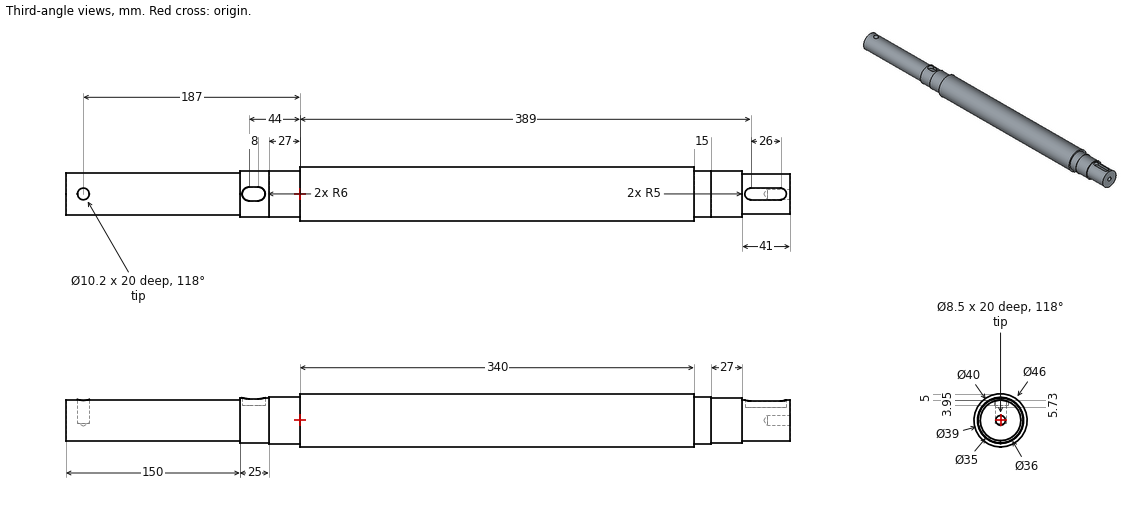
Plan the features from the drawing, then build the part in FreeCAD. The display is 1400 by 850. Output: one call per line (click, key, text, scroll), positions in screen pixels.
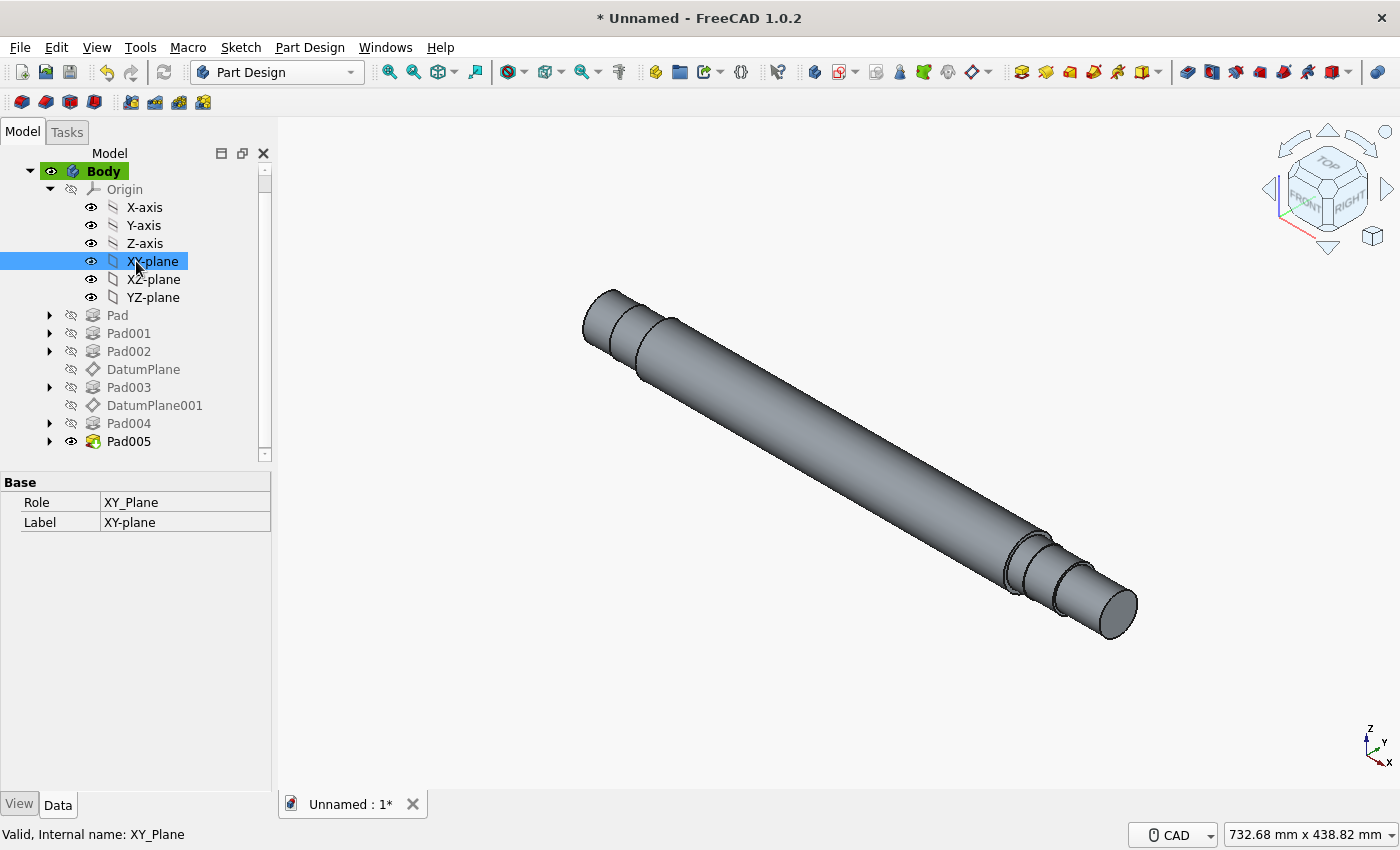
click(972, 72)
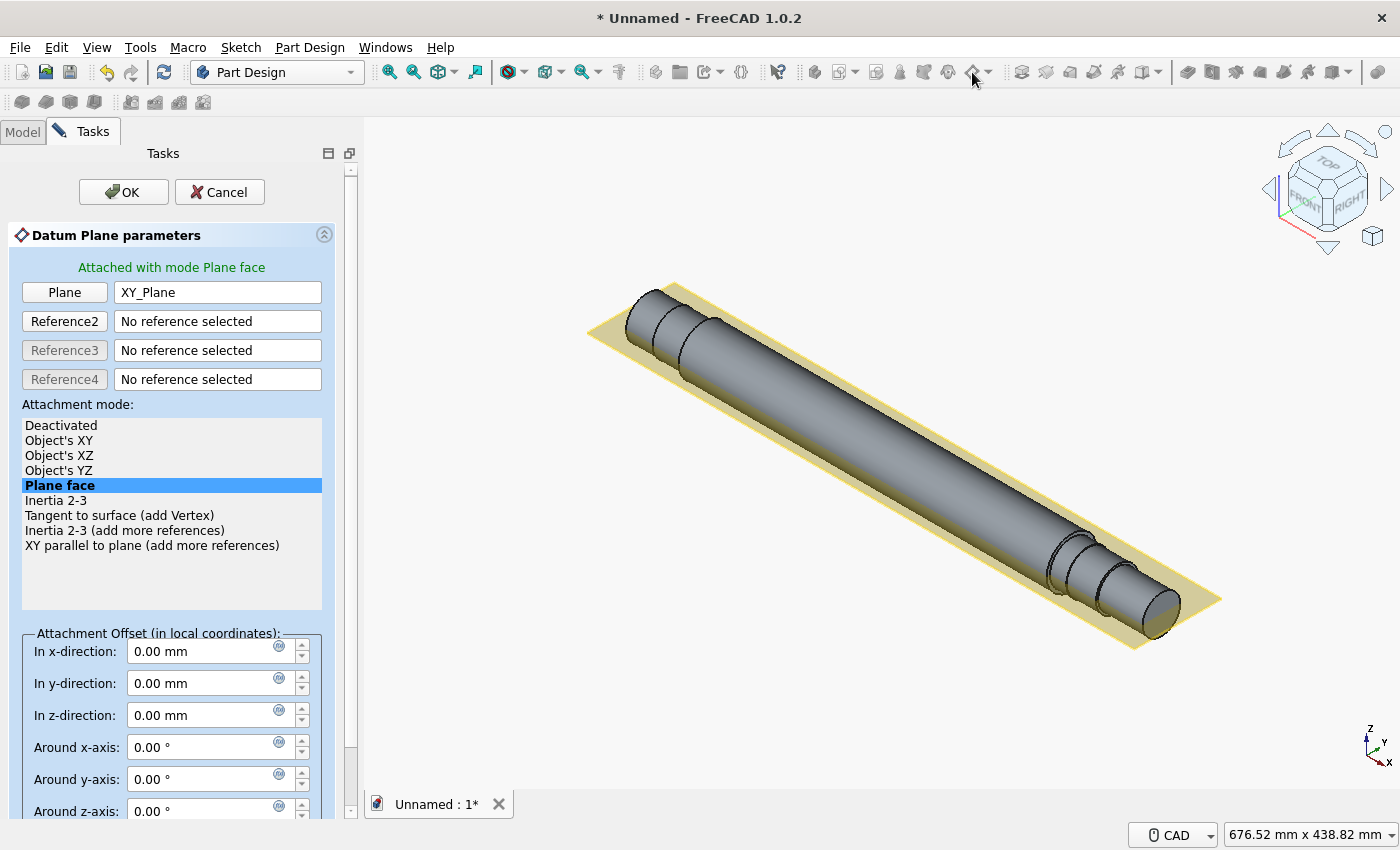
triple_click(210, 715)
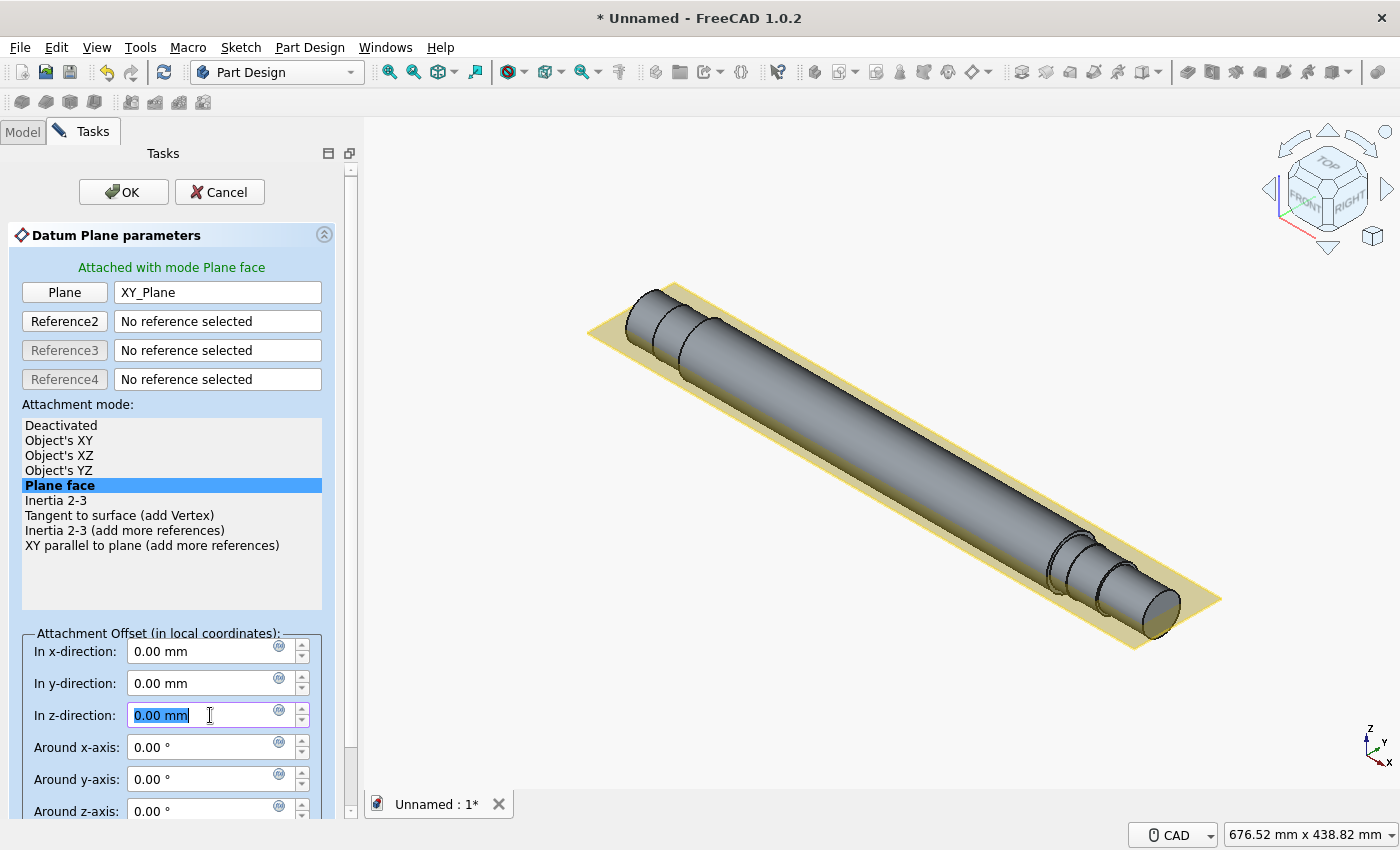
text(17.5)
key(Tab)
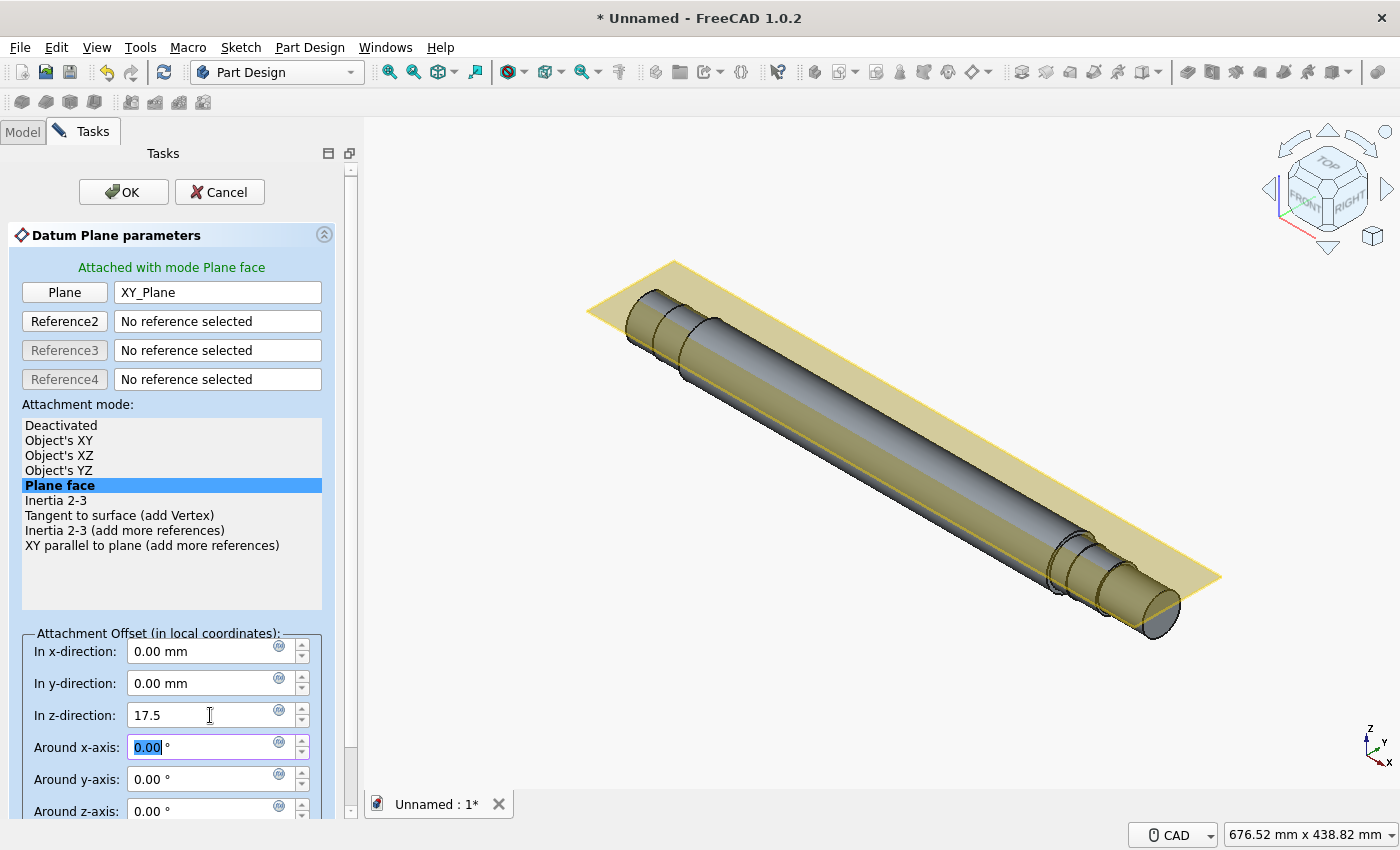
click(124, 192)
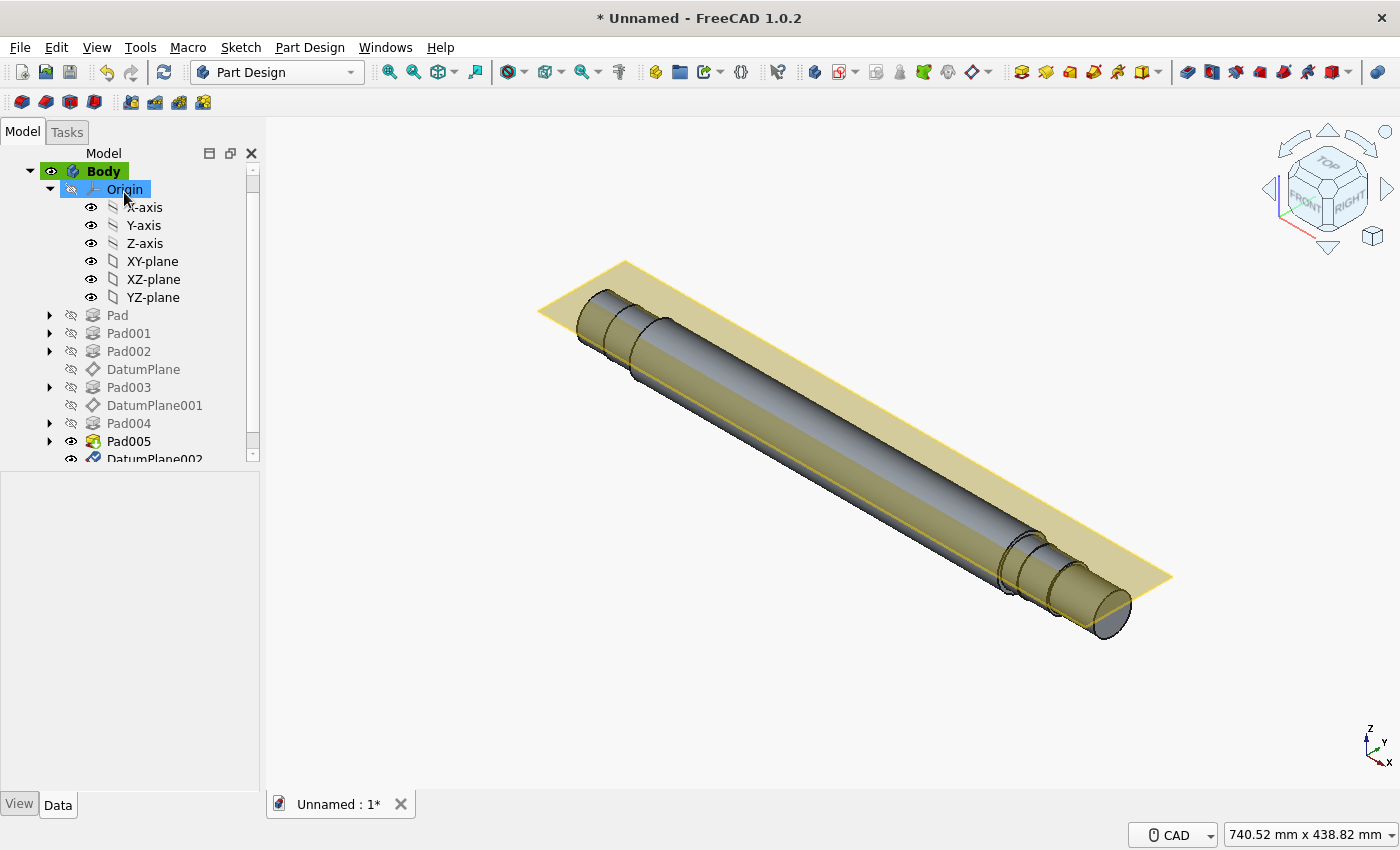
click(116, 459)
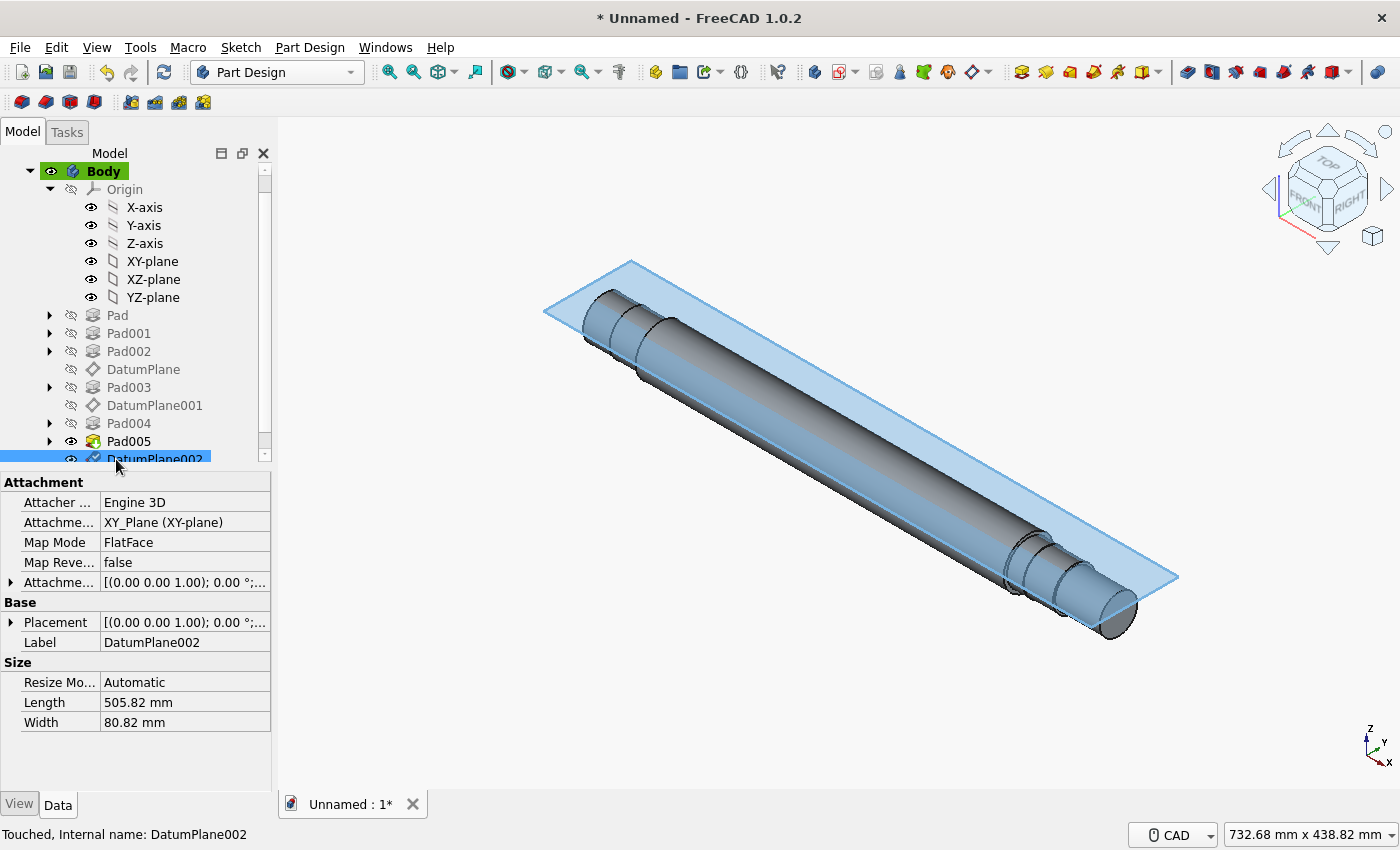
click(840, 72)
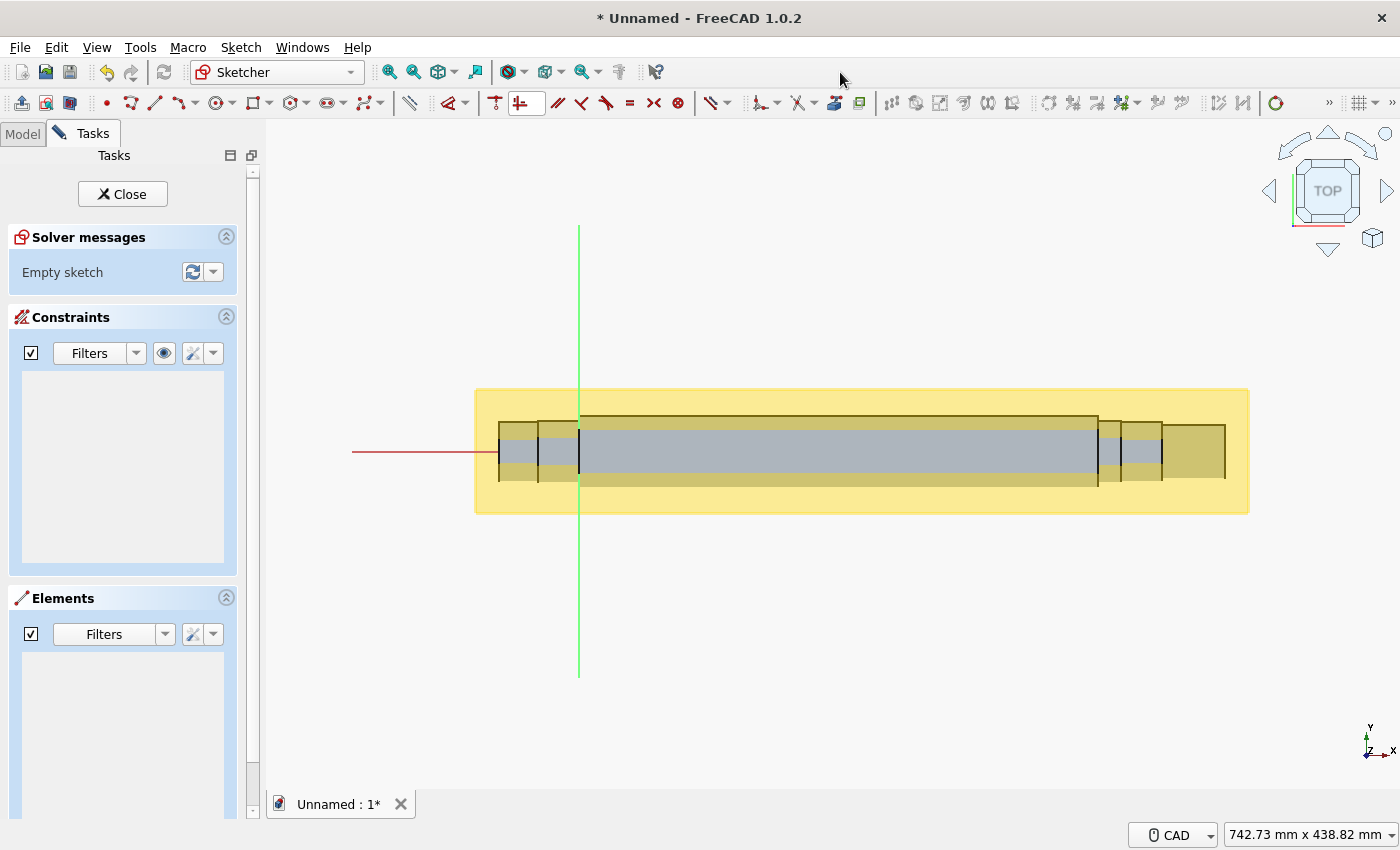
click(70, 104)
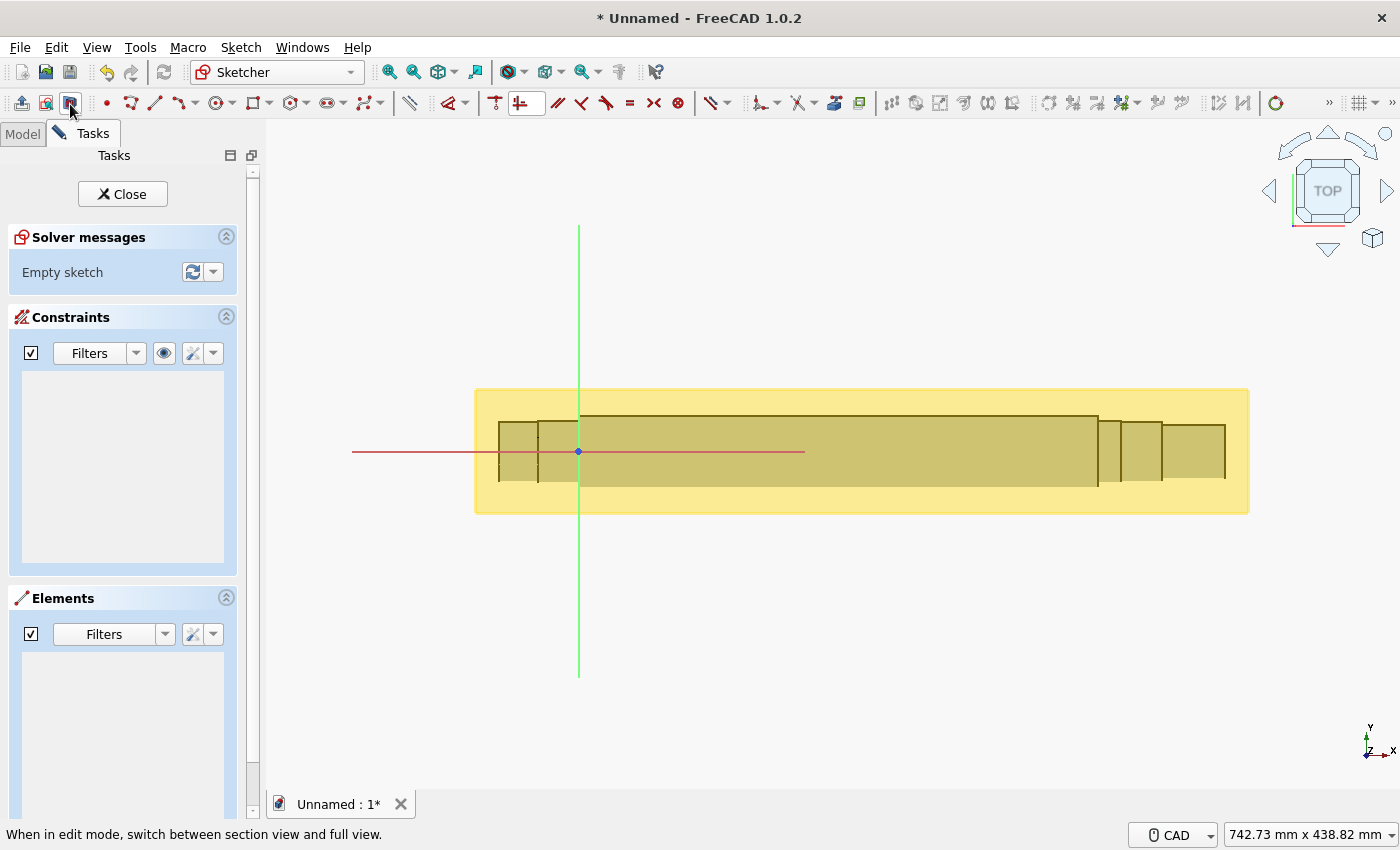
scroll(1235, 451, up, 12)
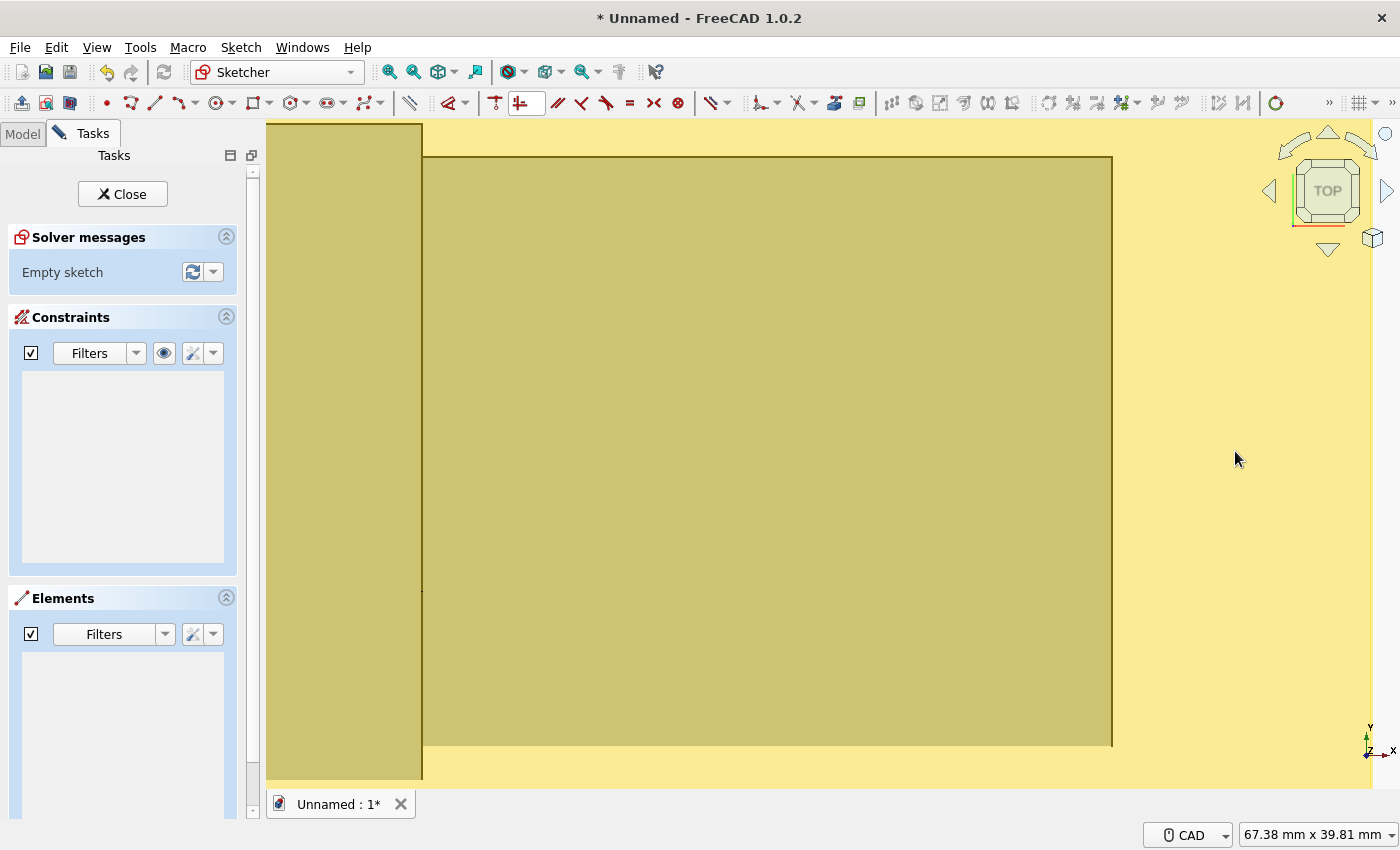
click(328, 104)